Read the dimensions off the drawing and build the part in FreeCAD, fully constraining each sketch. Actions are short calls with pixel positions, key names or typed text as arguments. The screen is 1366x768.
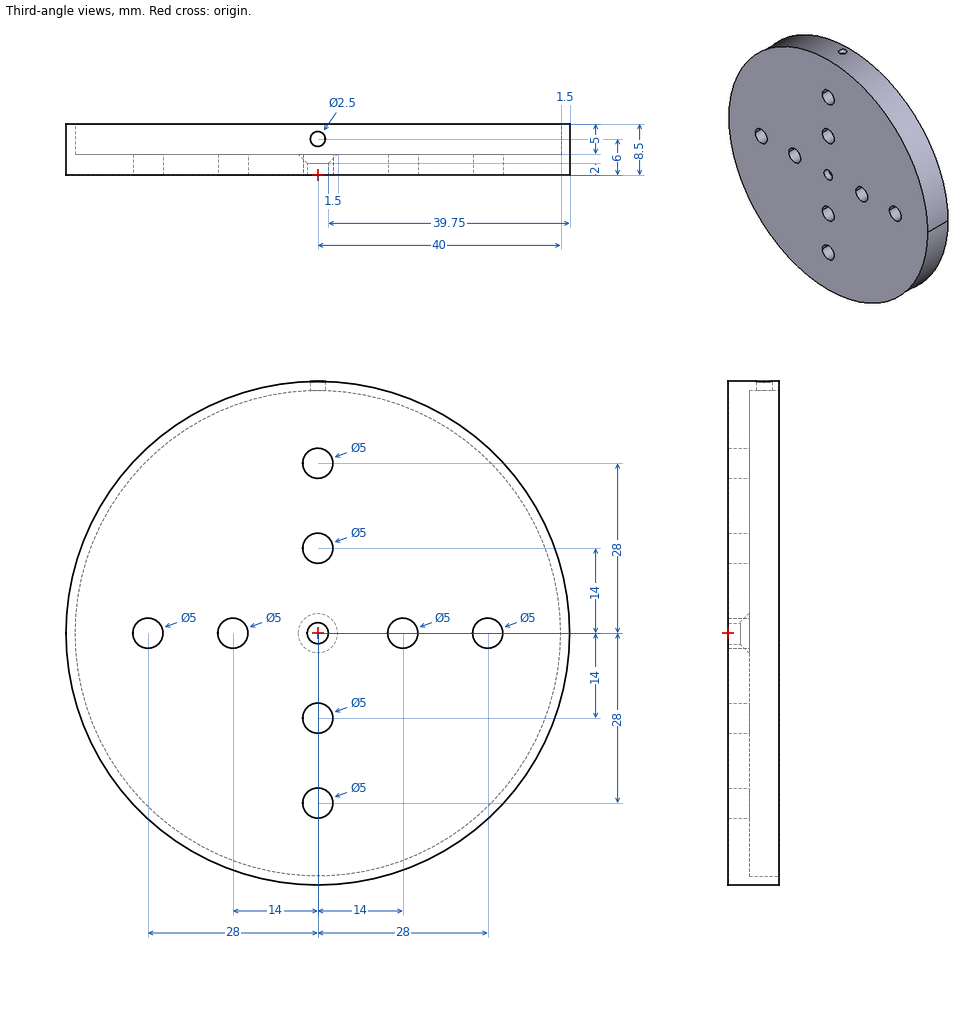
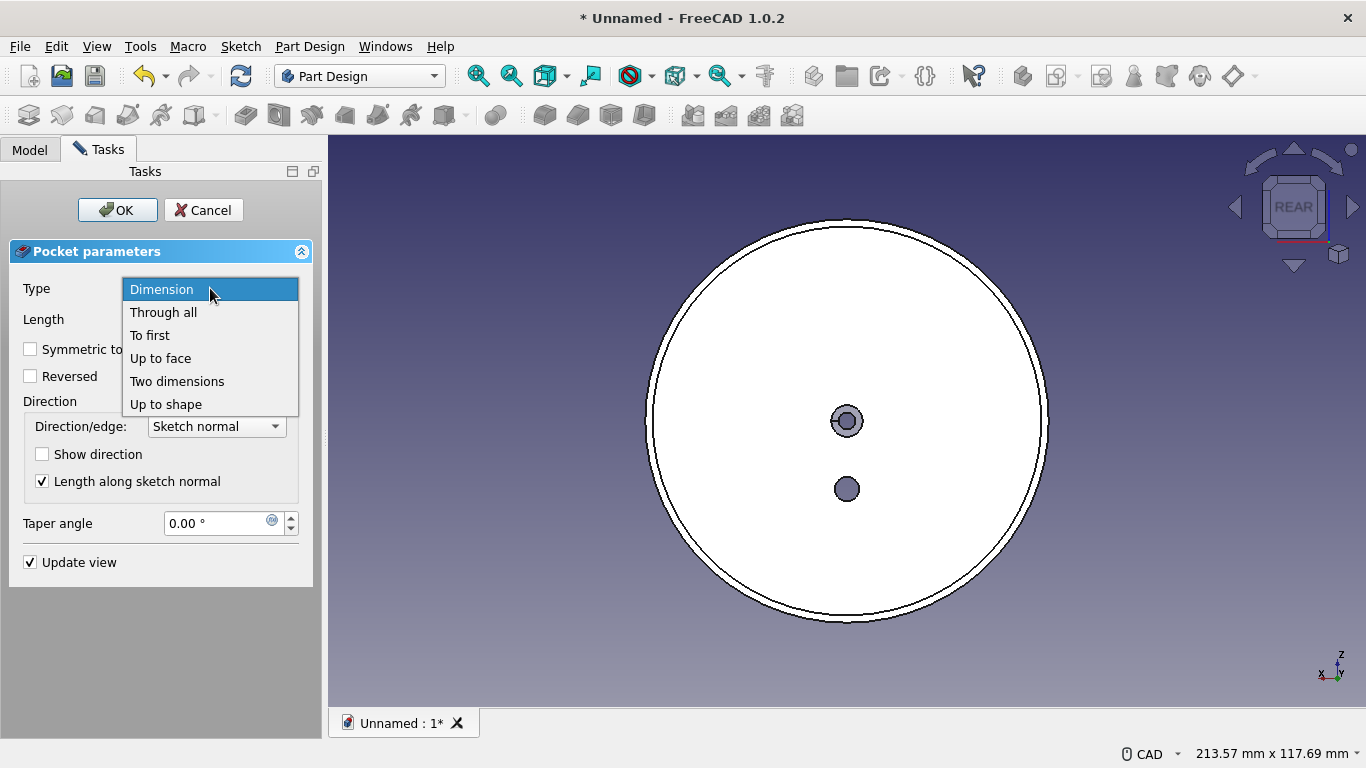
click(208, 336)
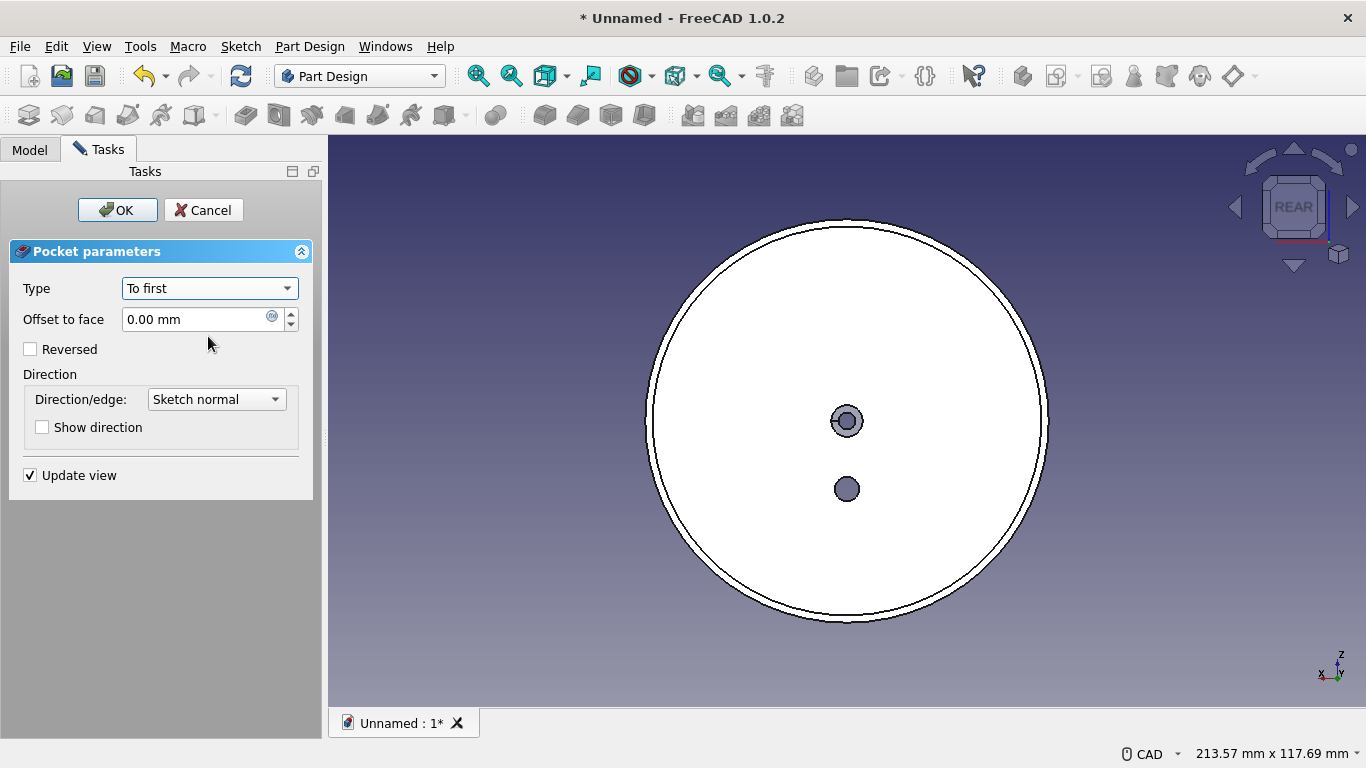
click(118, 210)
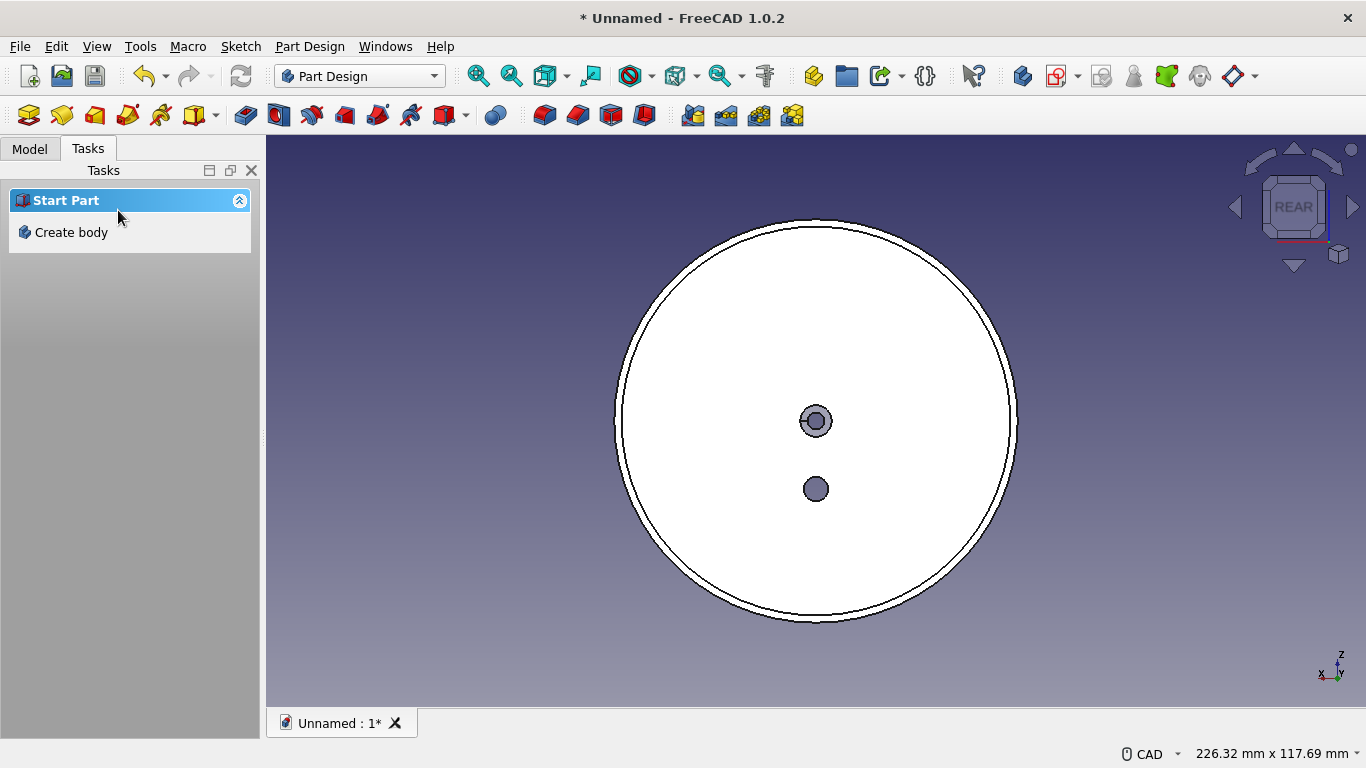
click(705, 420)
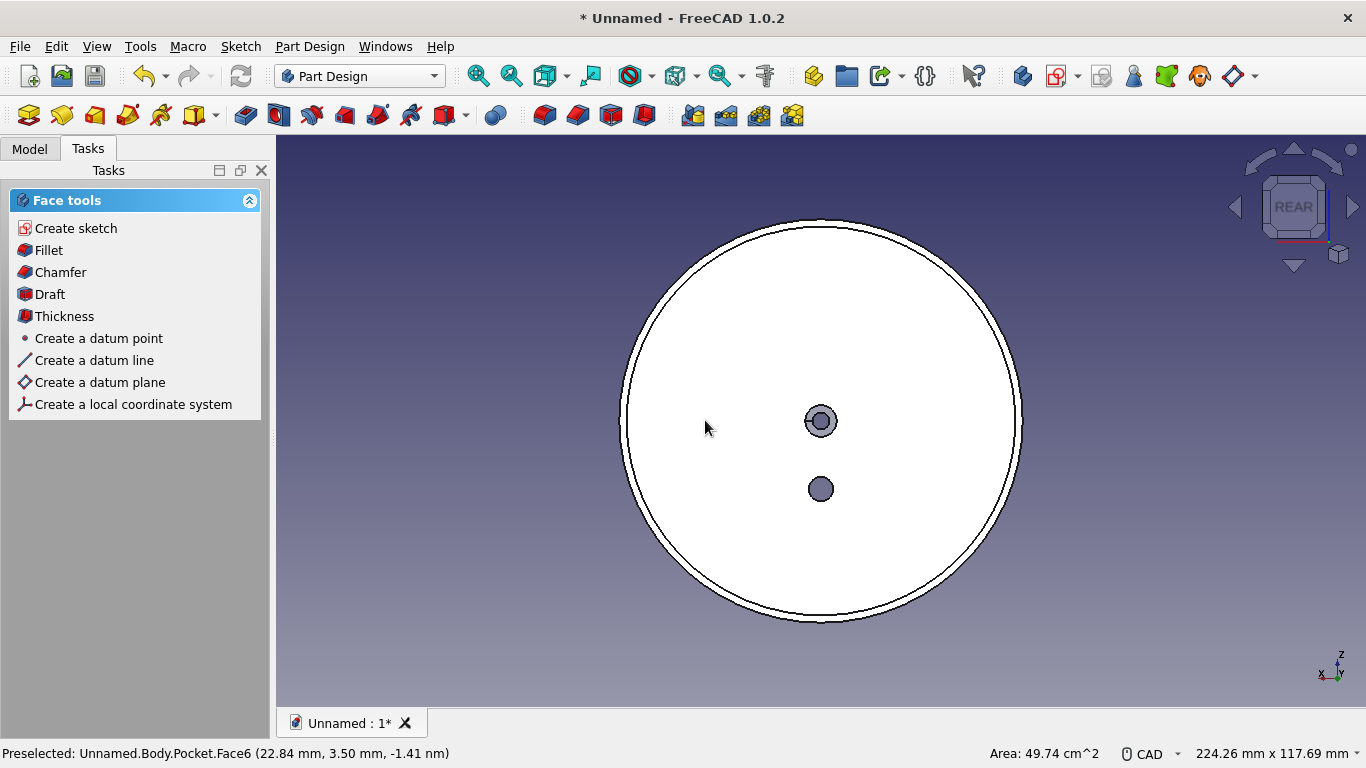
click(1056, 76)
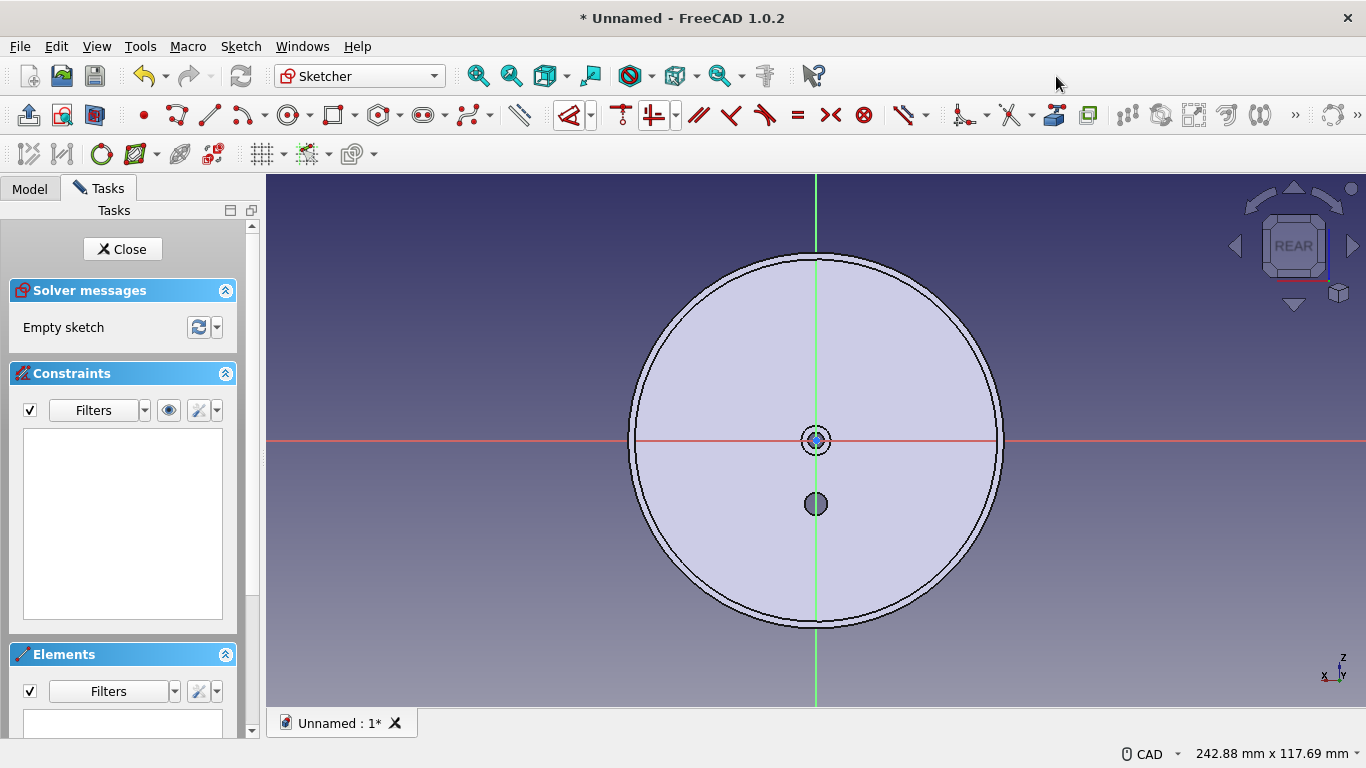
click(95, 116)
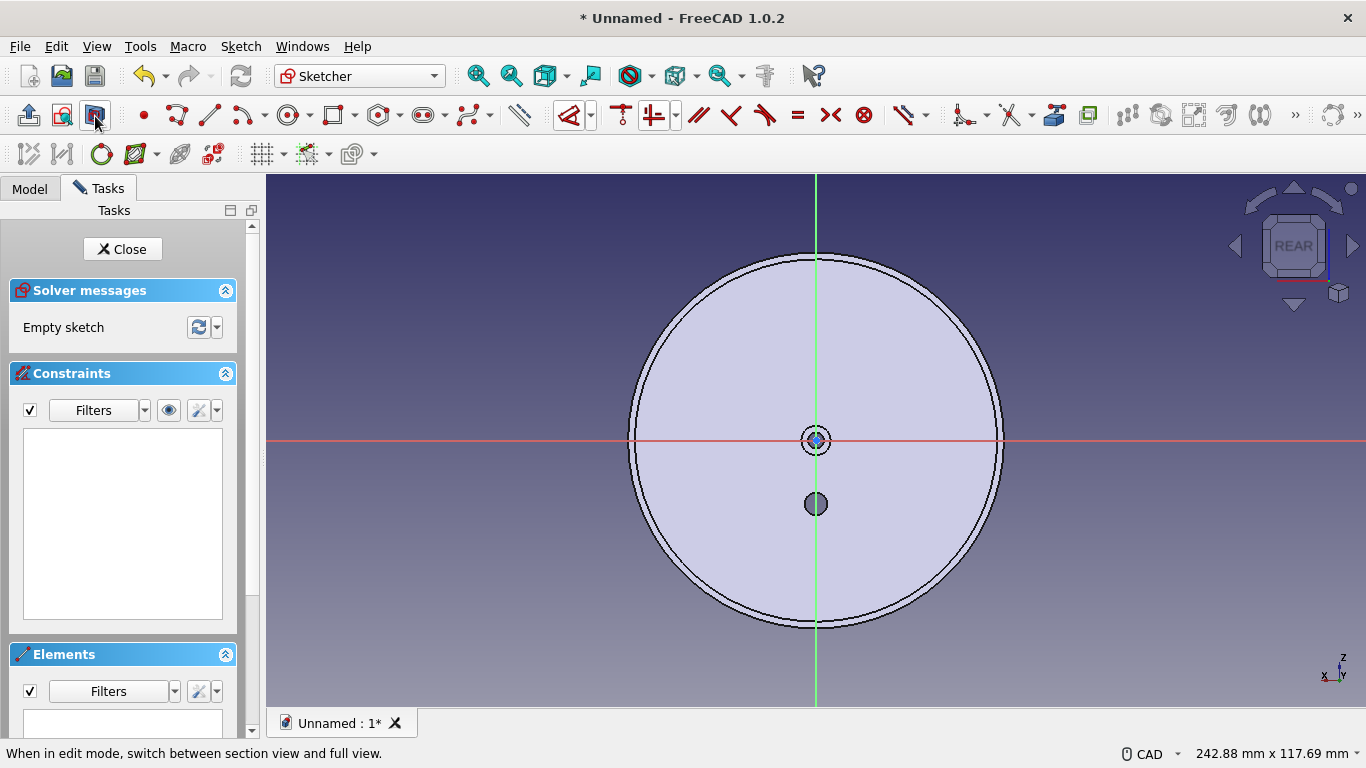
scroll(753, 441, up, 13)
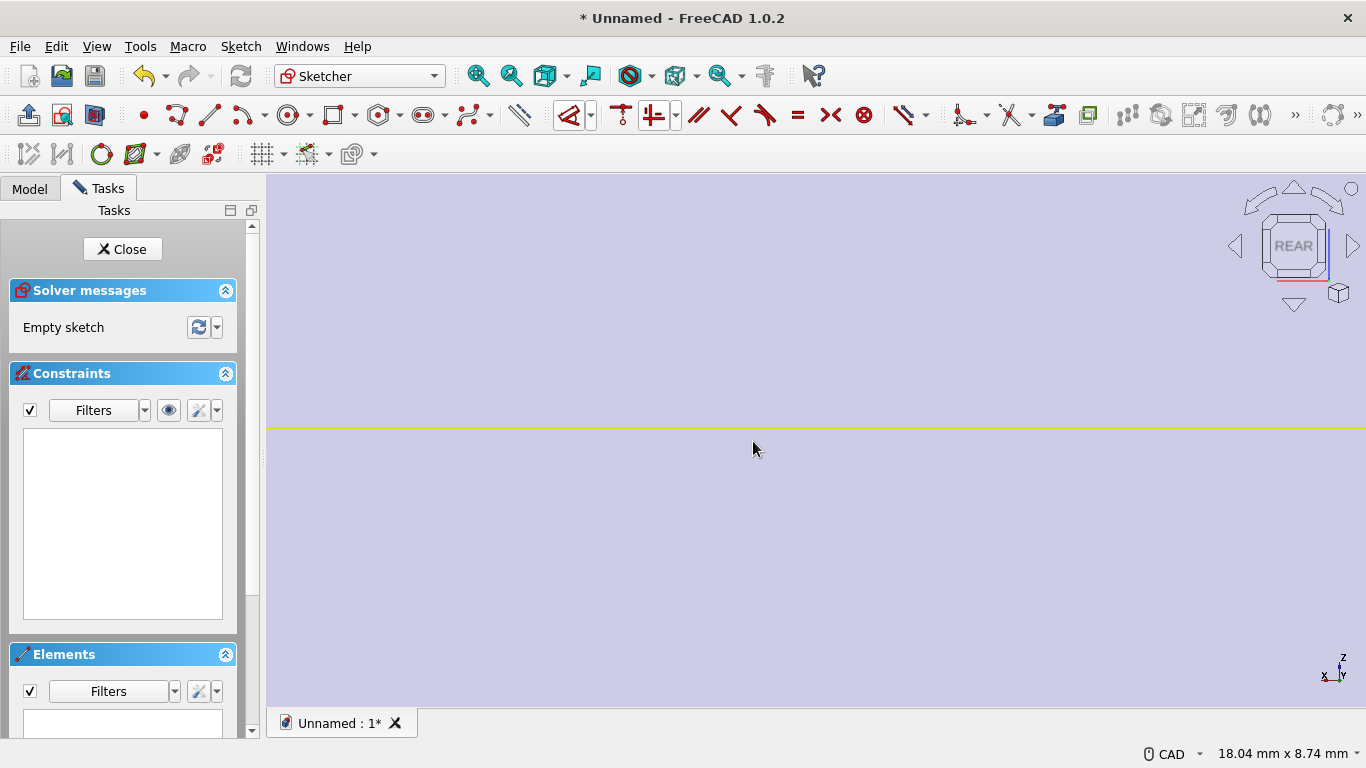
click(288, 116)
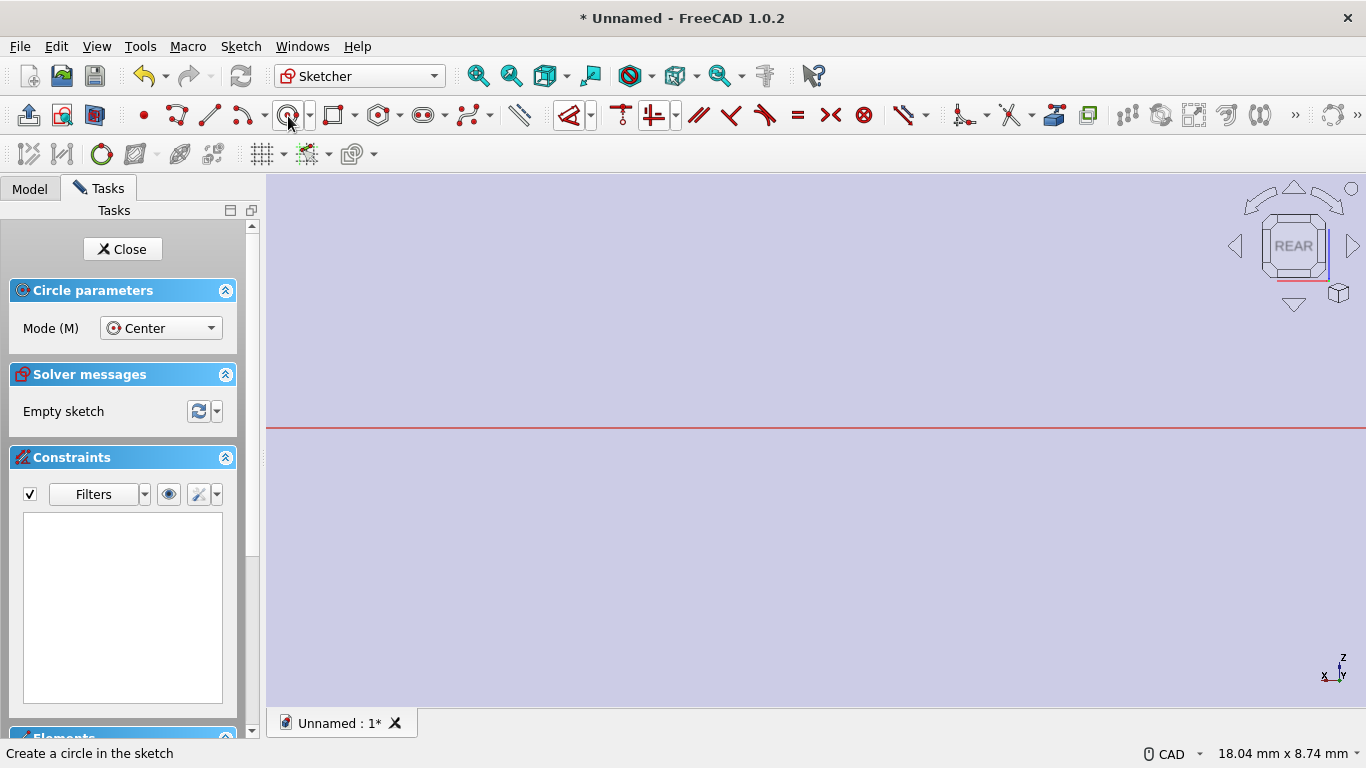
click(742, 428)
click(850, 320)
key(Escape)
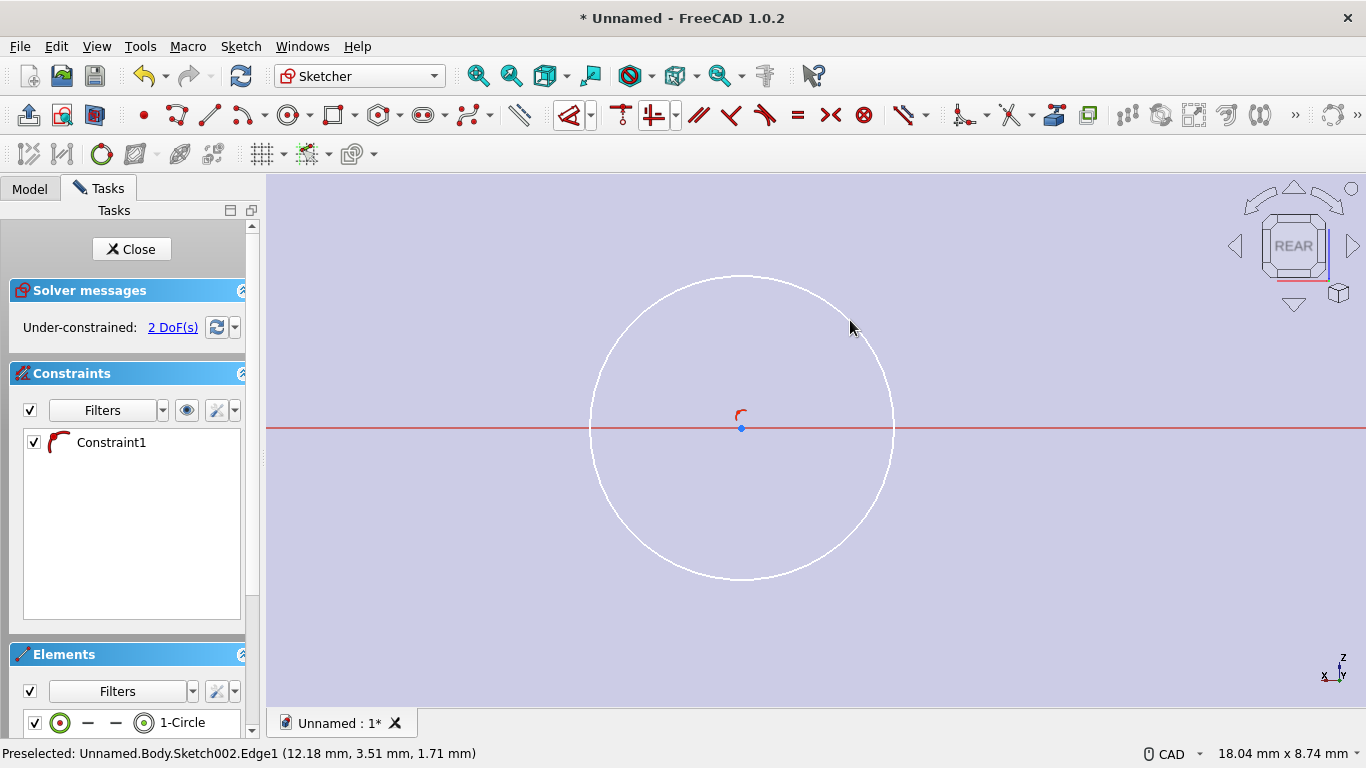
click(849, 320)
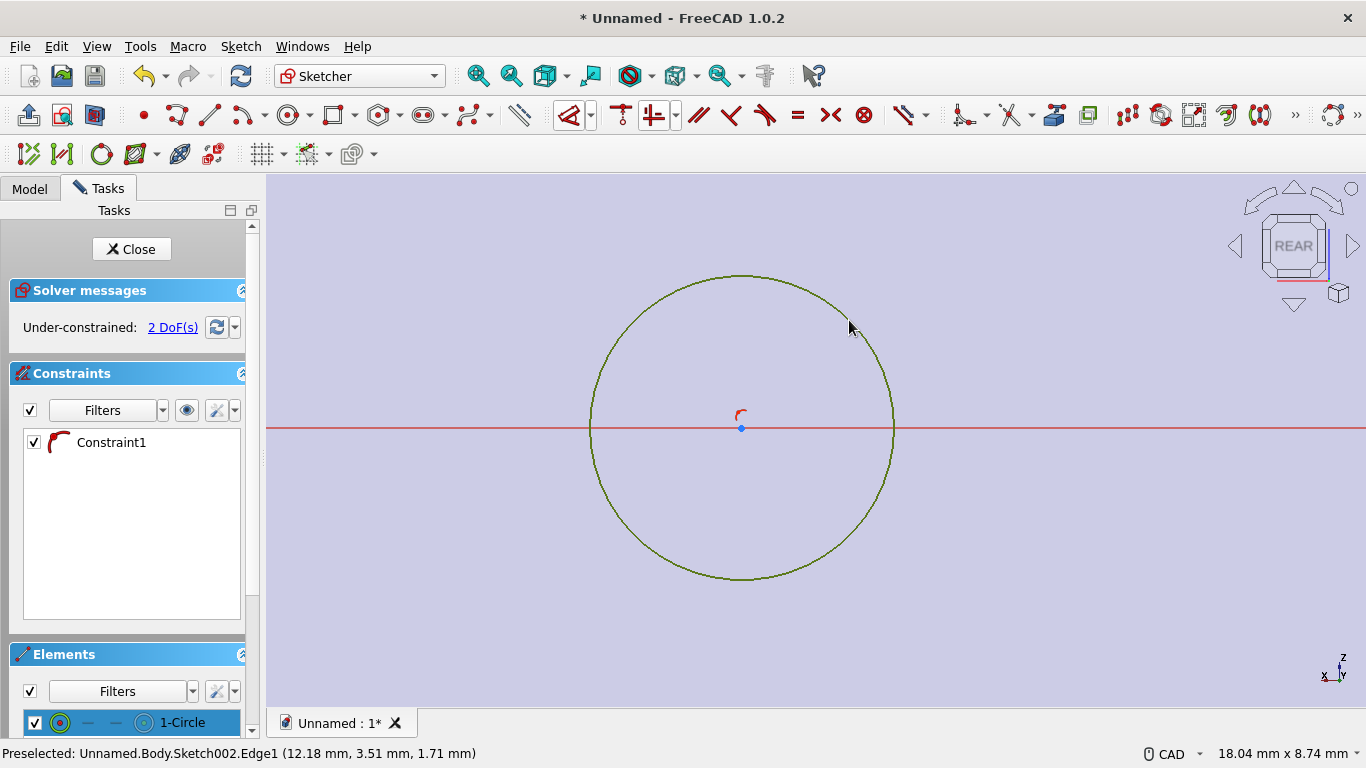
click(590, 116)